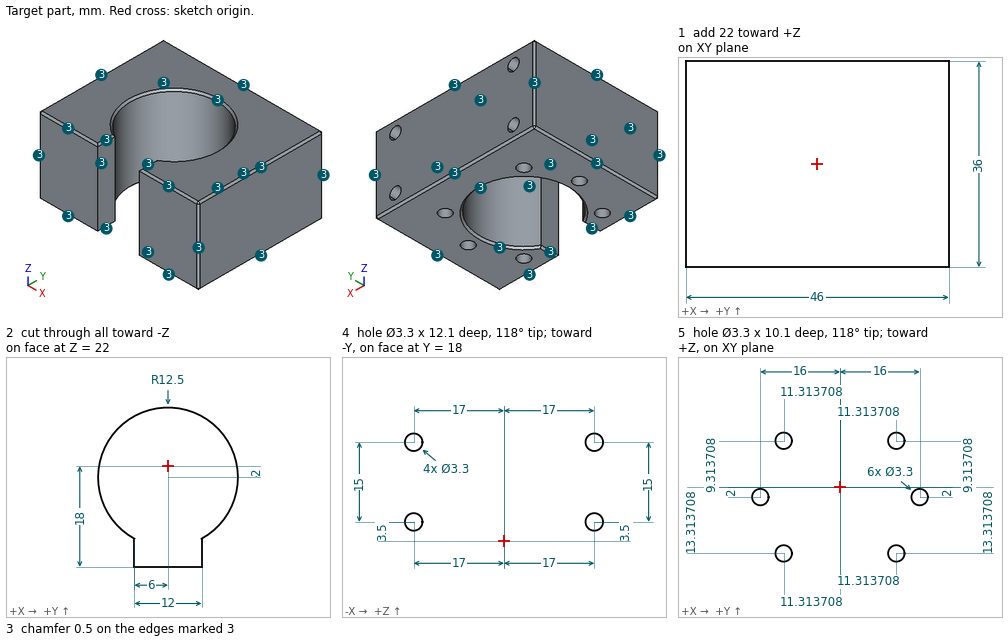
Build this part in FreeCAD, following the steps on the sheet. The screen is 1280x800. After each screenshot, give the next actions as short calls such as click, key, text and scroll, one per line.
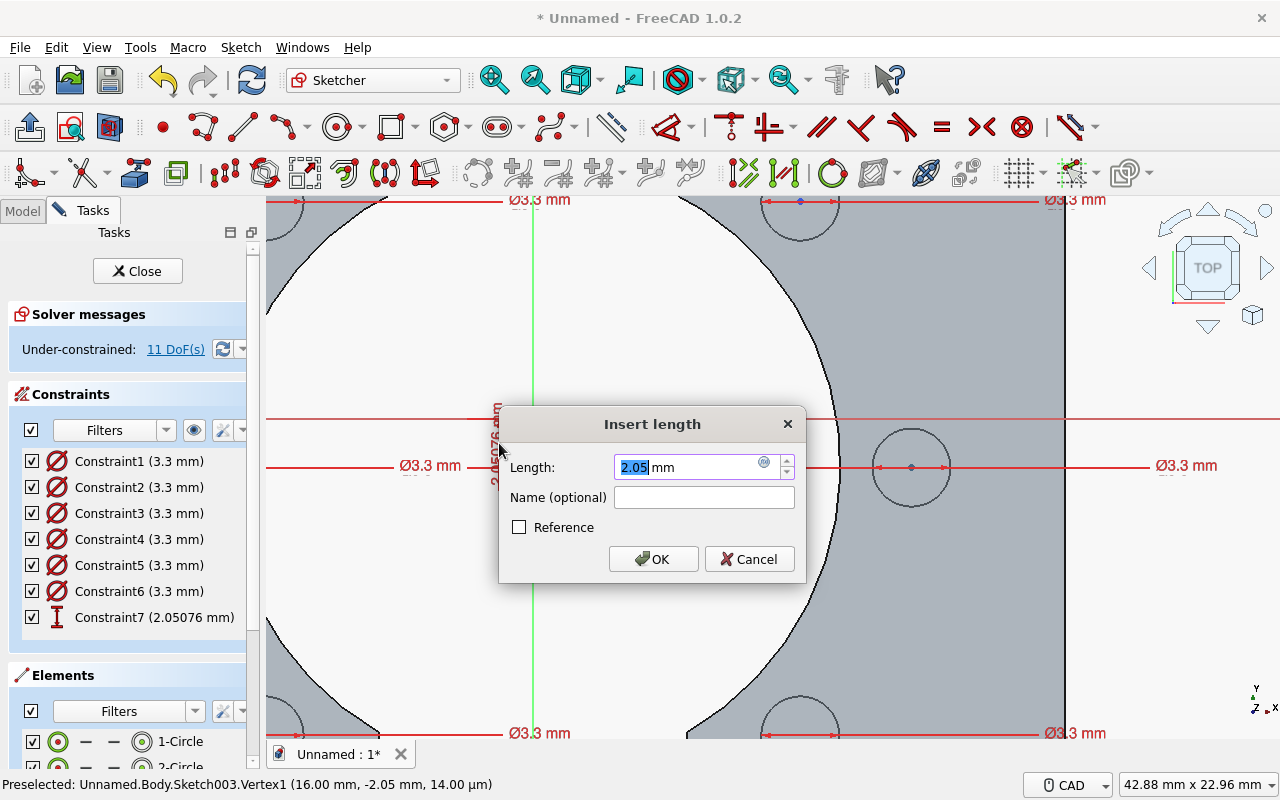
text(2)
key(Return)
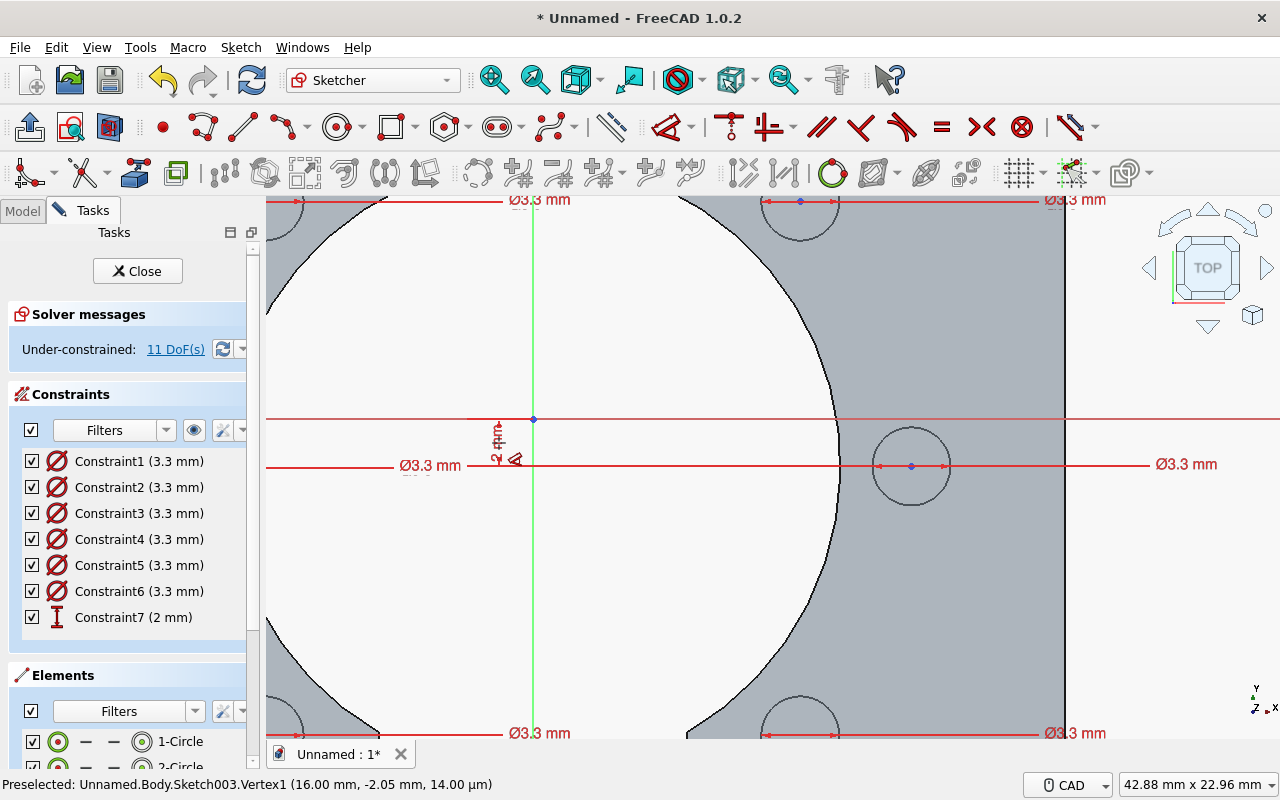
scroll(913, 469, down, 3)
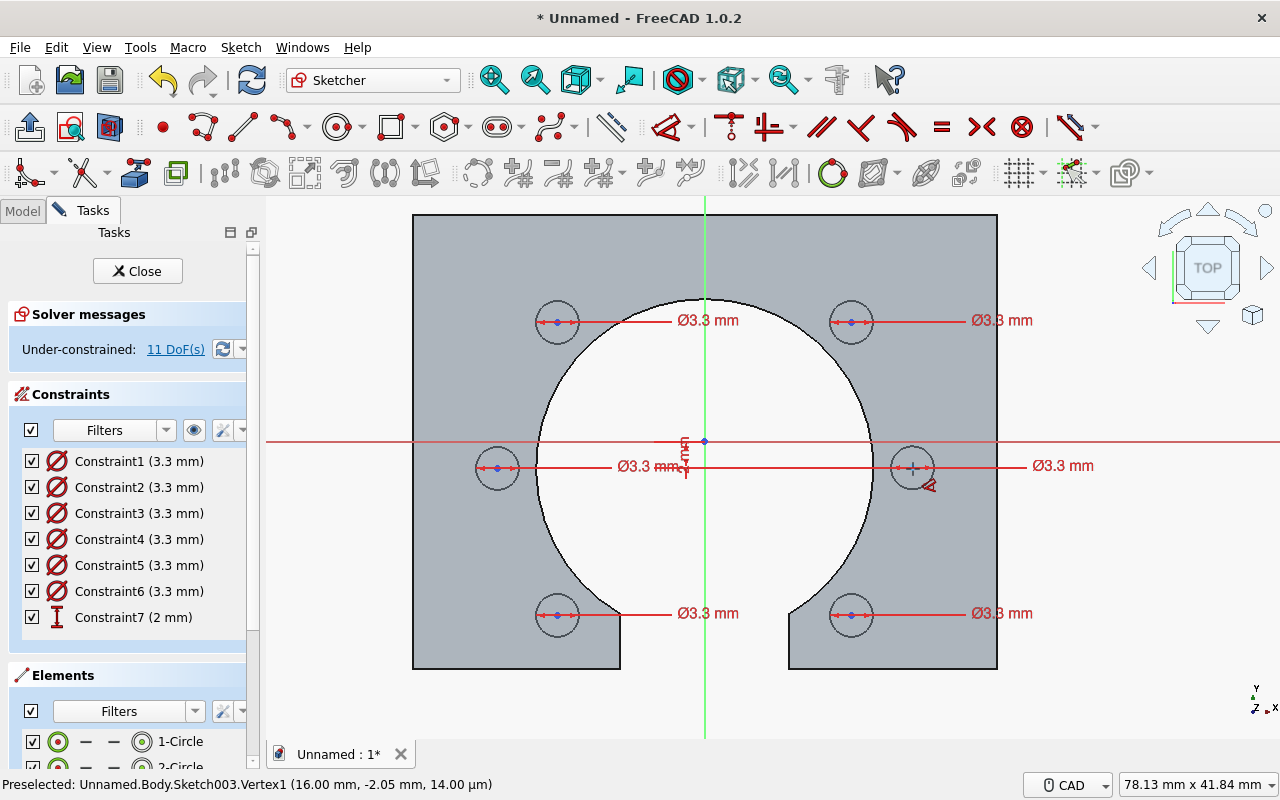
scroll(497, 468, up, 3)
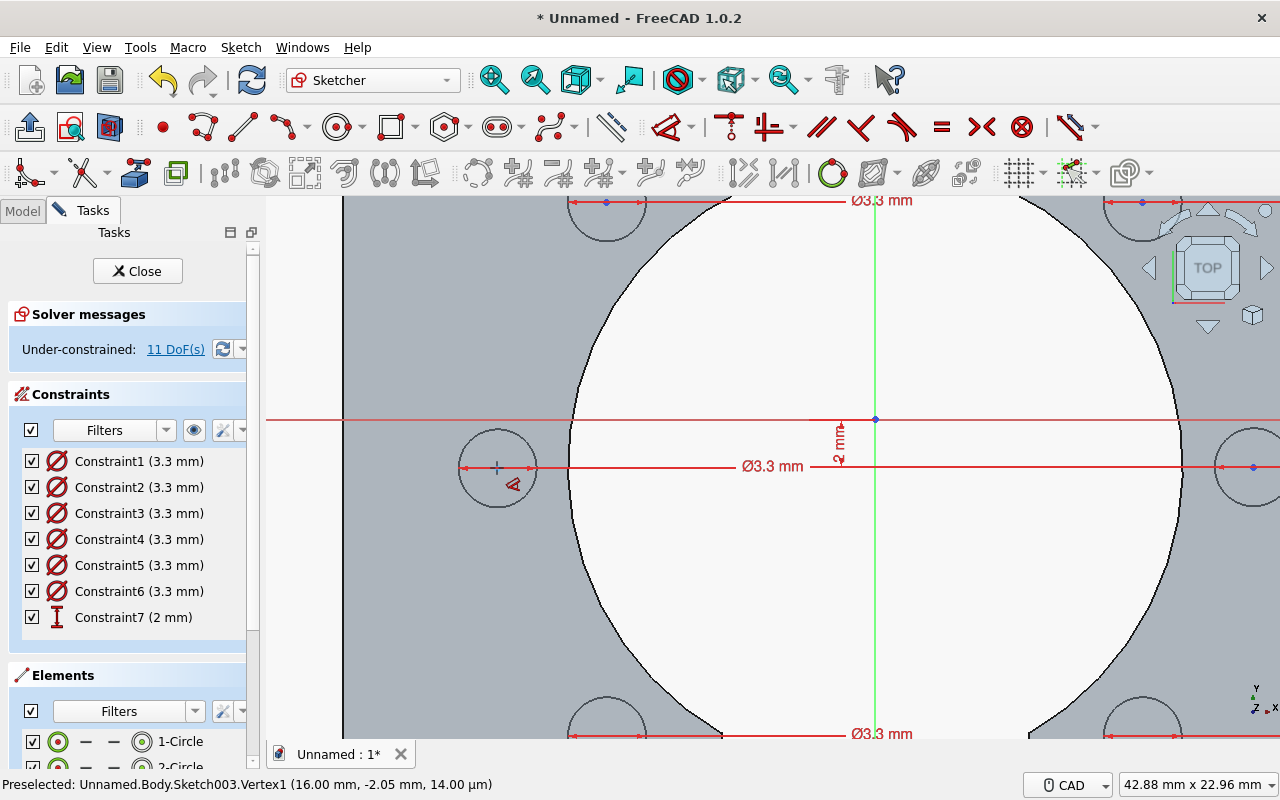
click(498, 468)
click(440, 444)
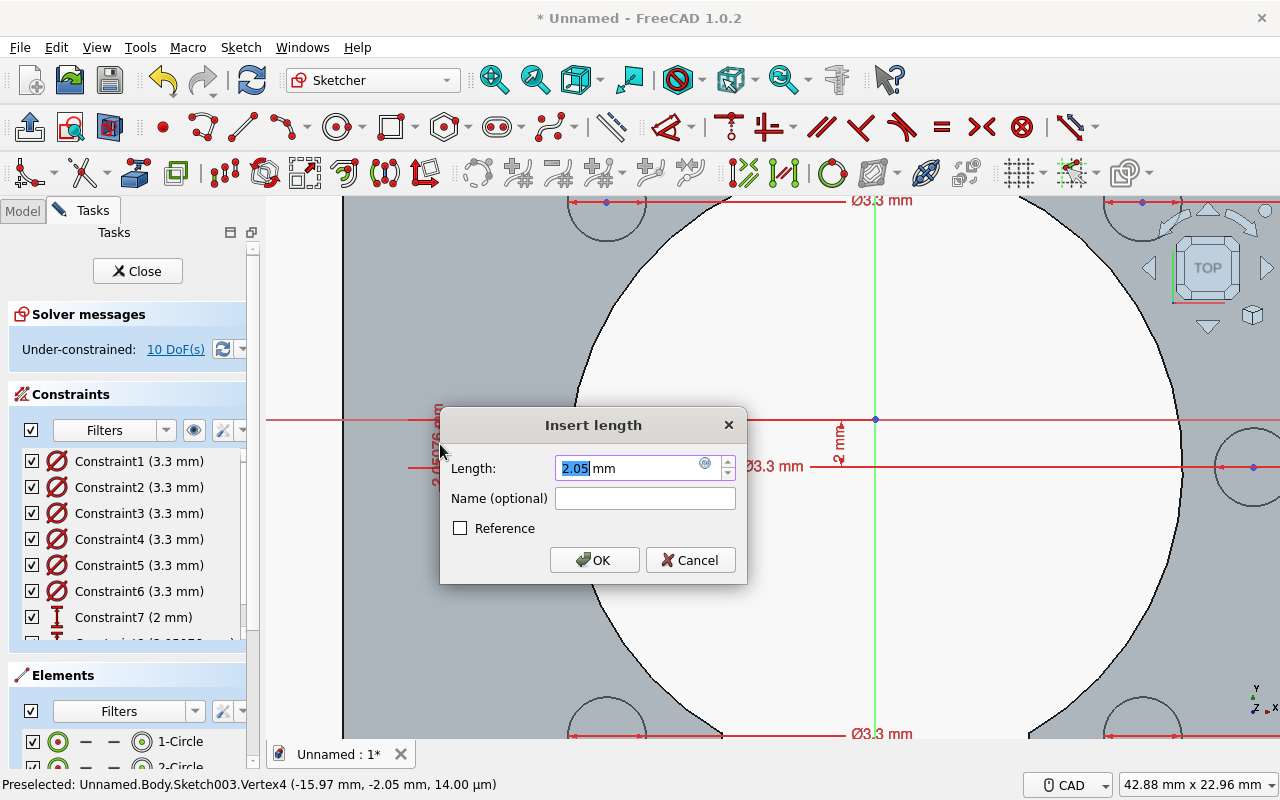
text(2)
key(Return)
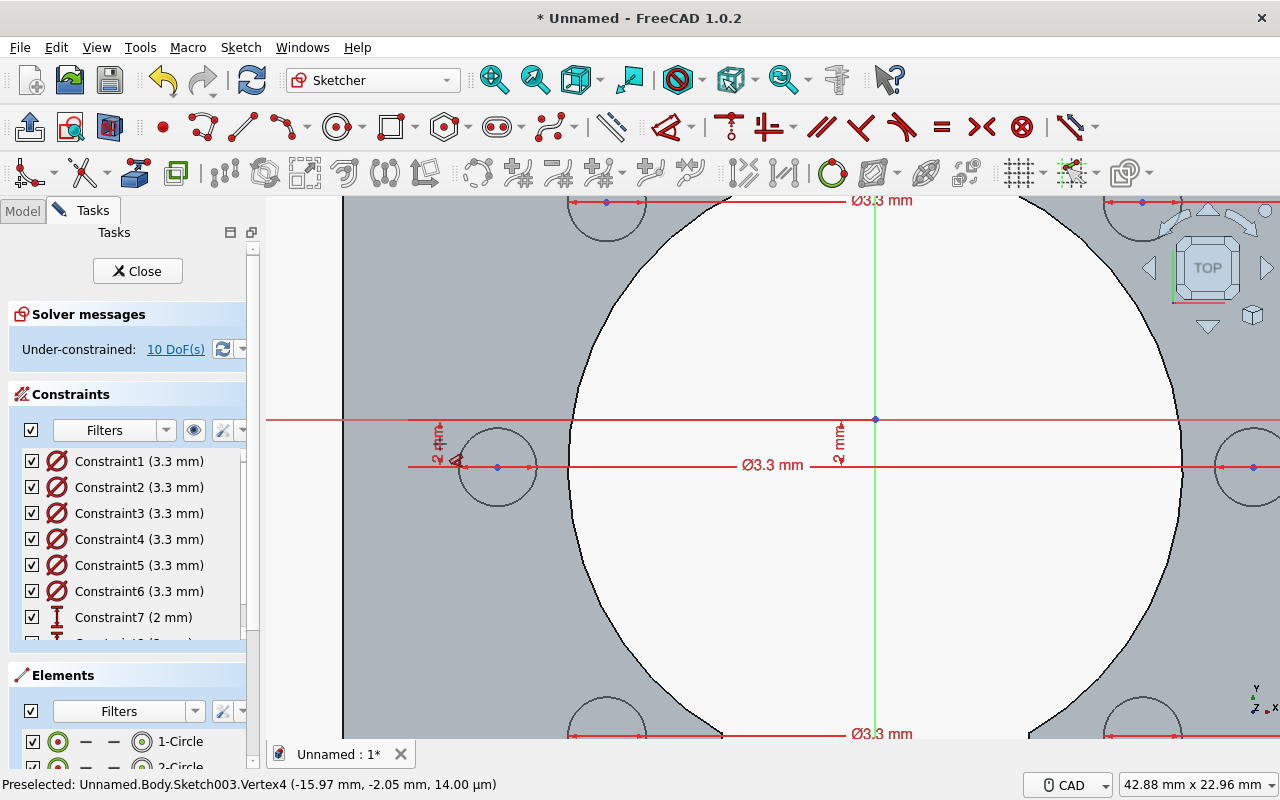
scroll(497, 468, down, 3)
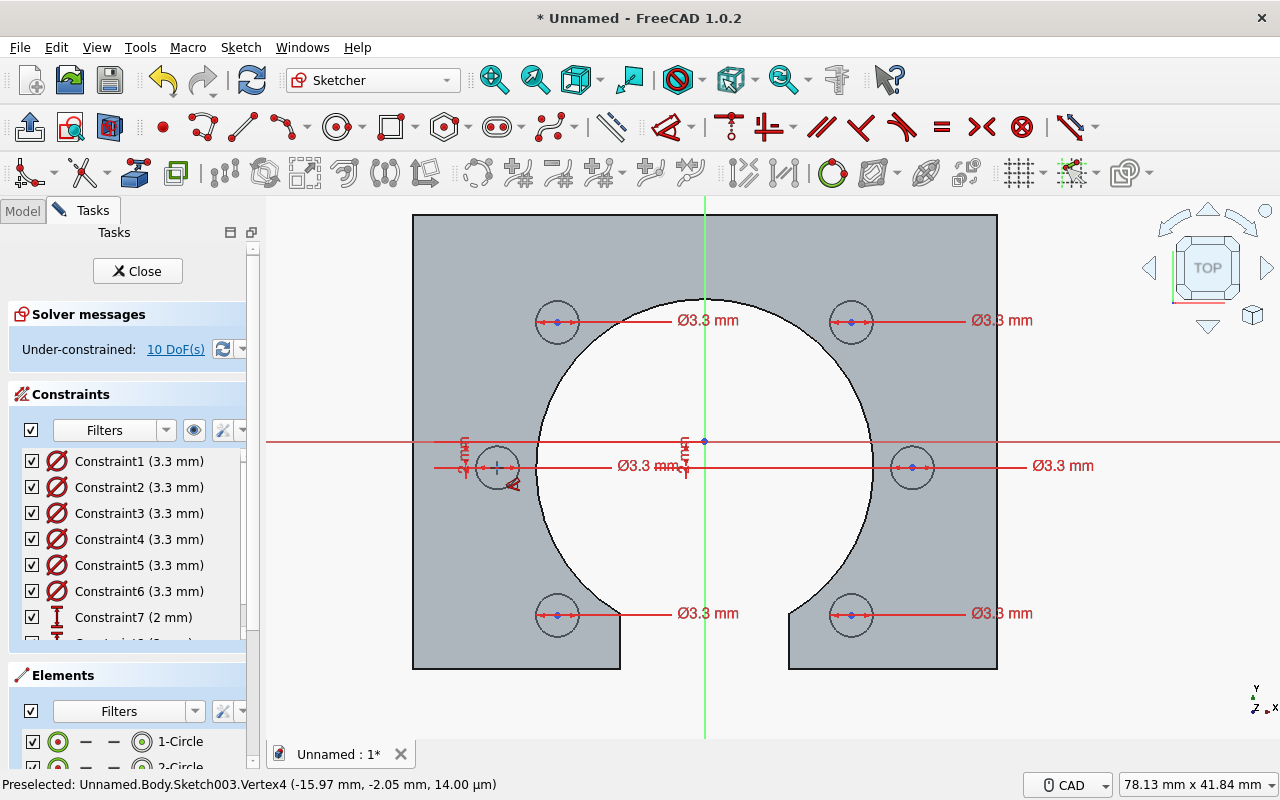
click(912, 468)
click(809, 408)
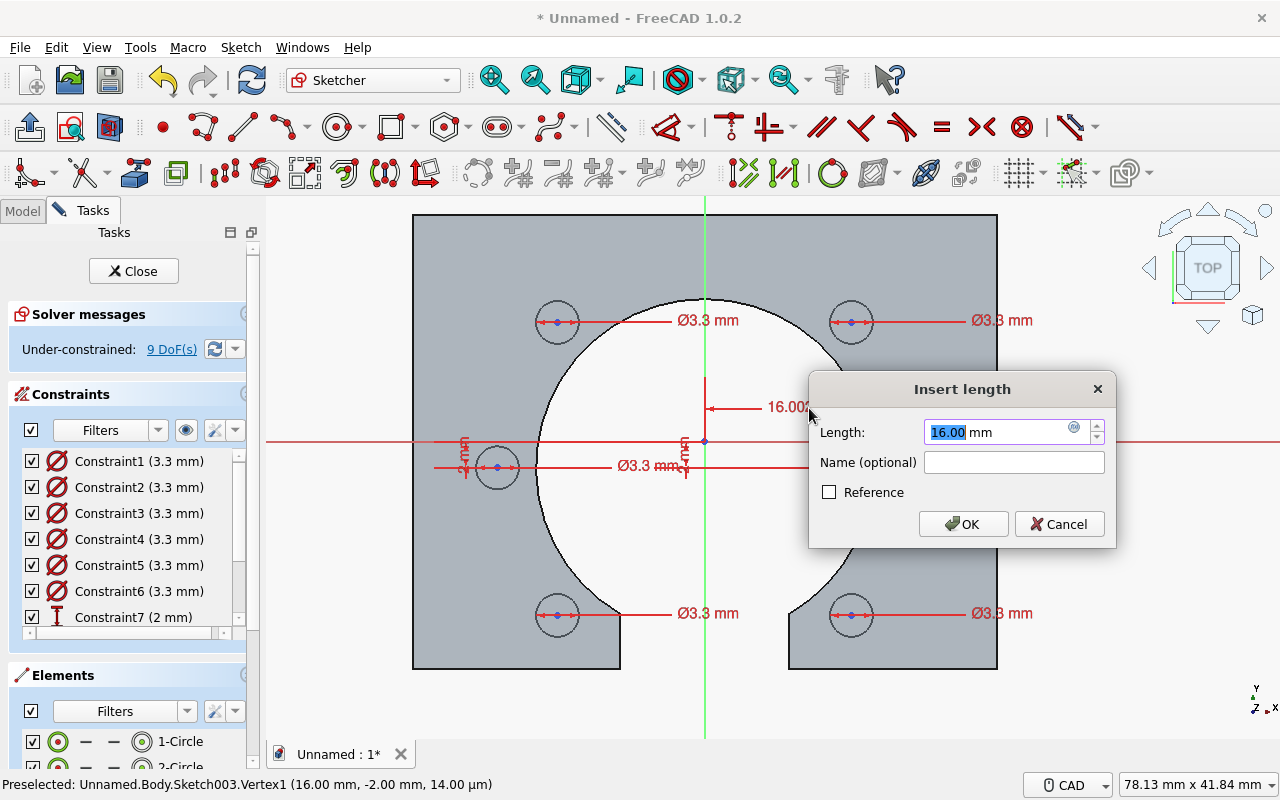
text(16)
key(Return)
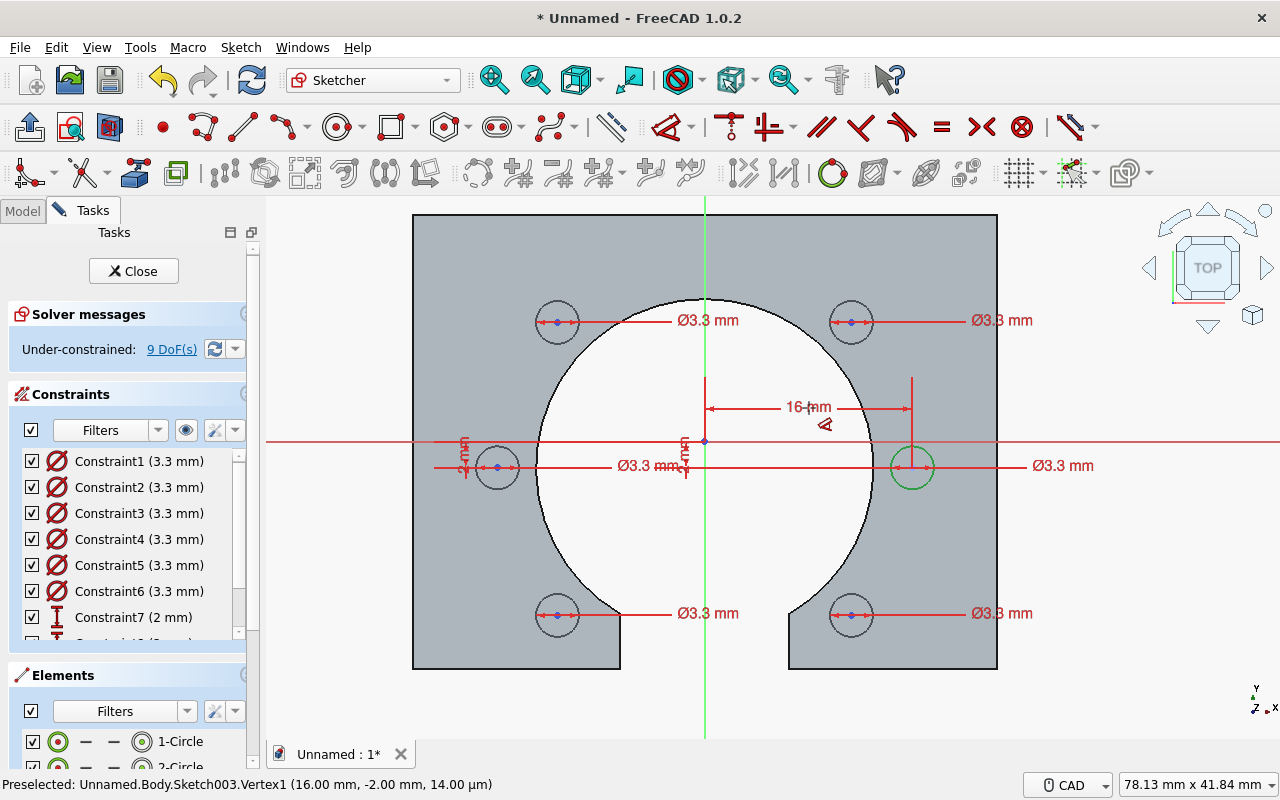
click(497, 468)
click(601, 408)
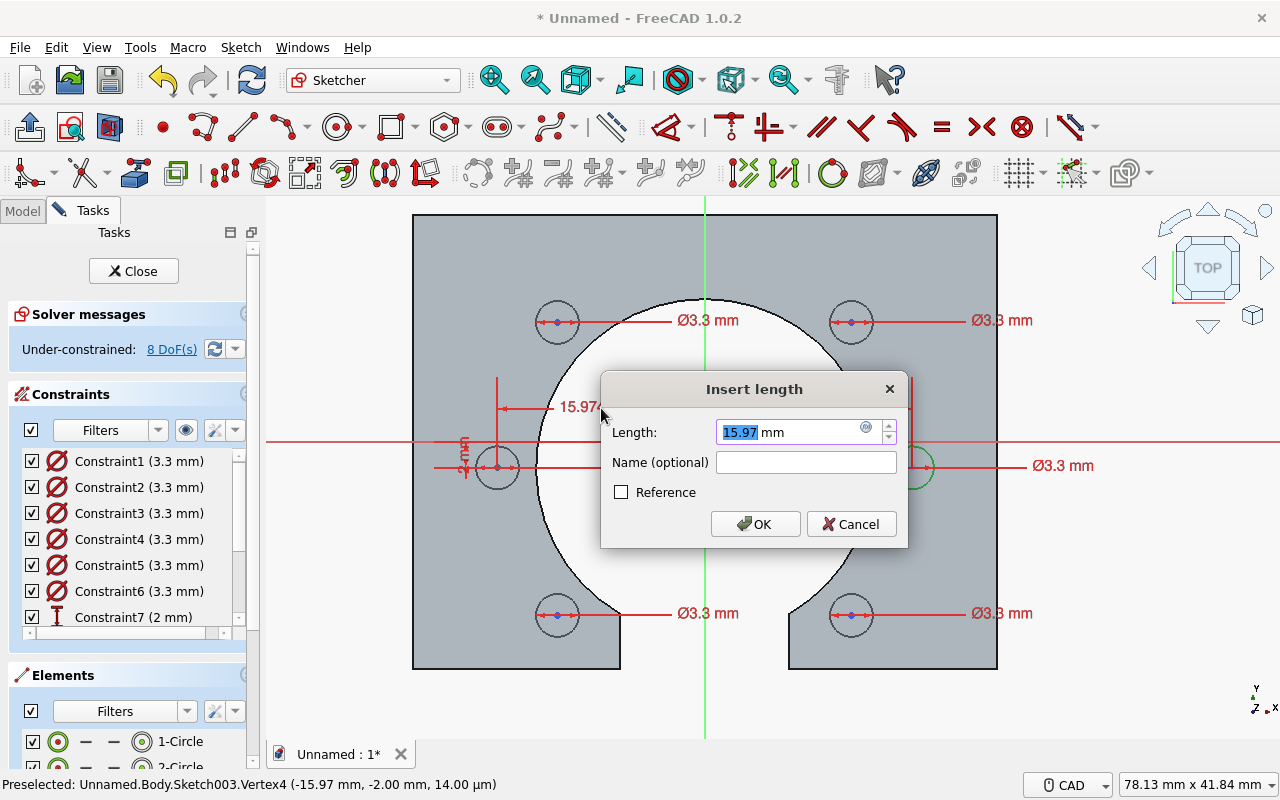
text(16)
key(Return)